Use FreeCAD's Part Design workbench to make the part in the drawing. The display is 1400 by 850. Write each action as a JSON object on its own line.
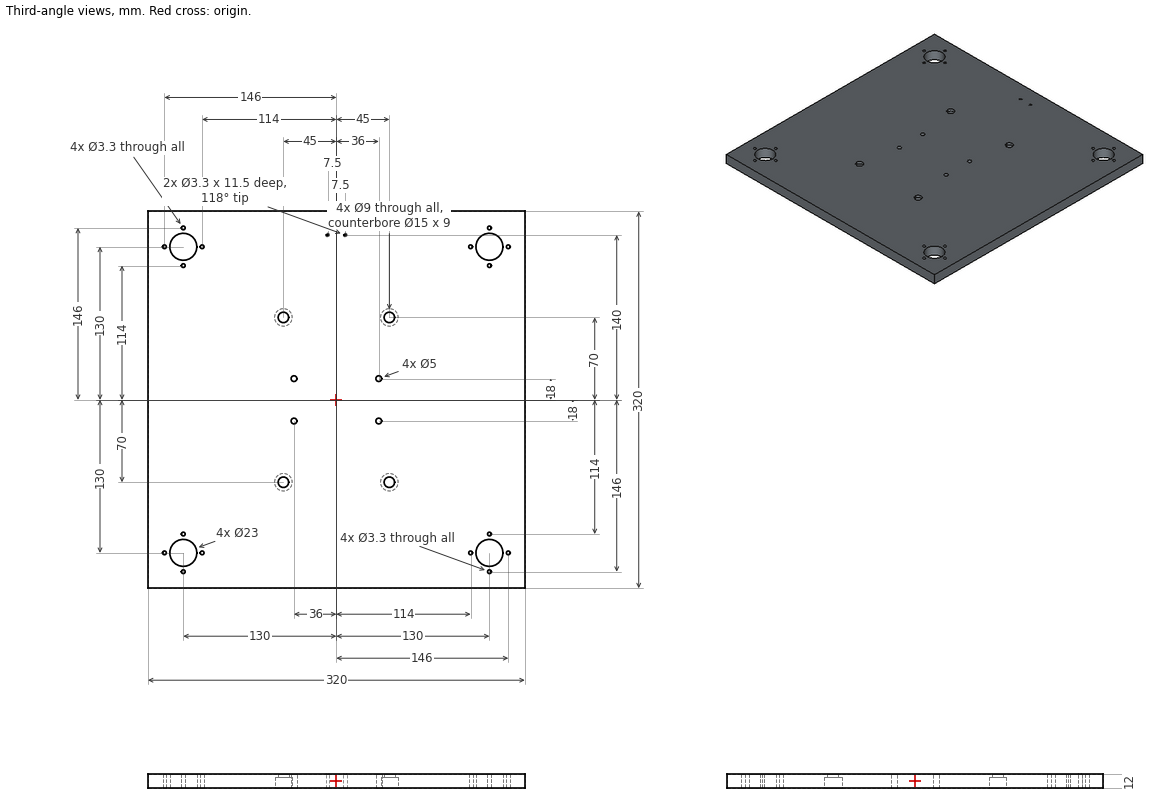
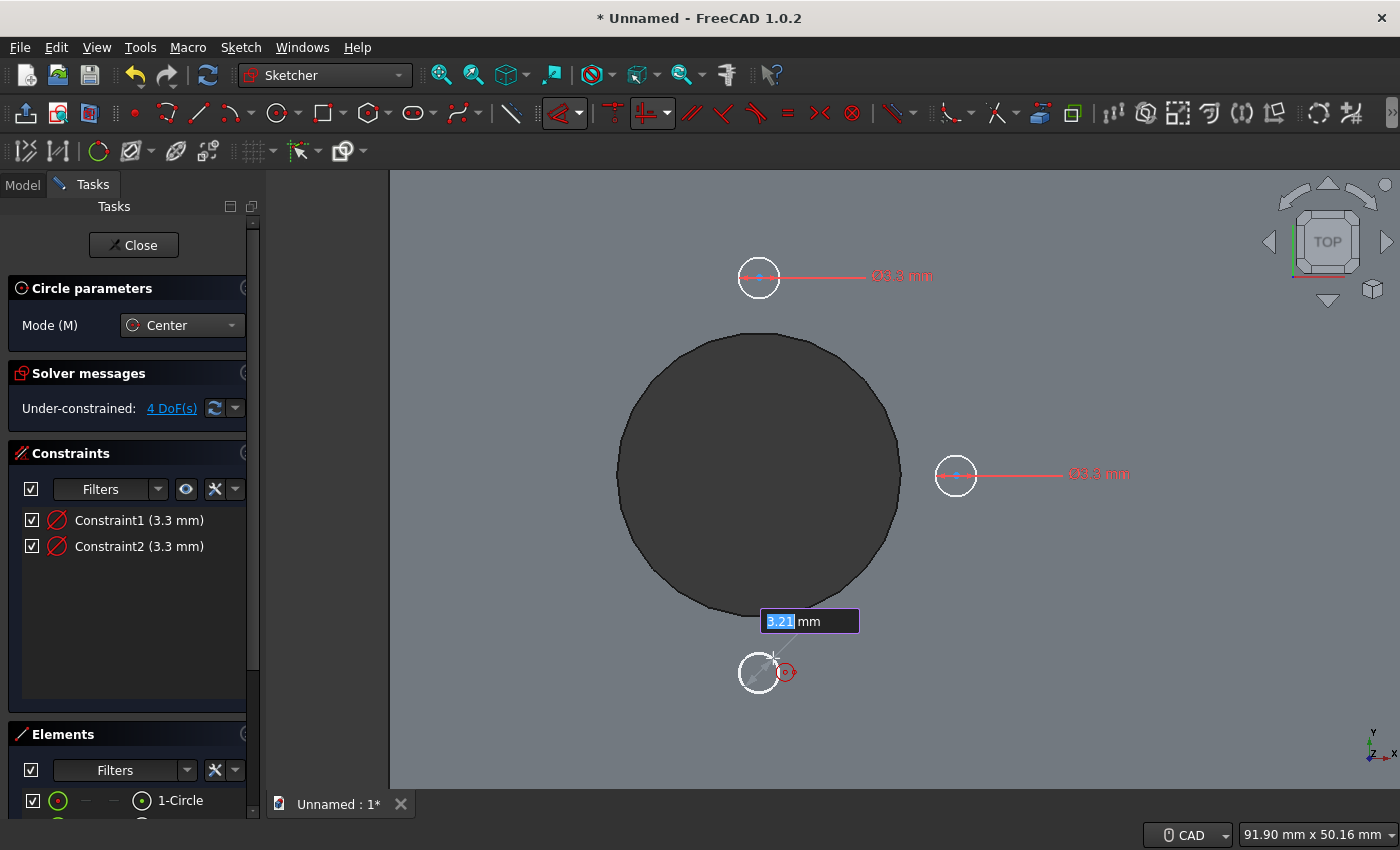
{"action": "type", "text": "3.3"}
{"action": "key", "text": "Return"}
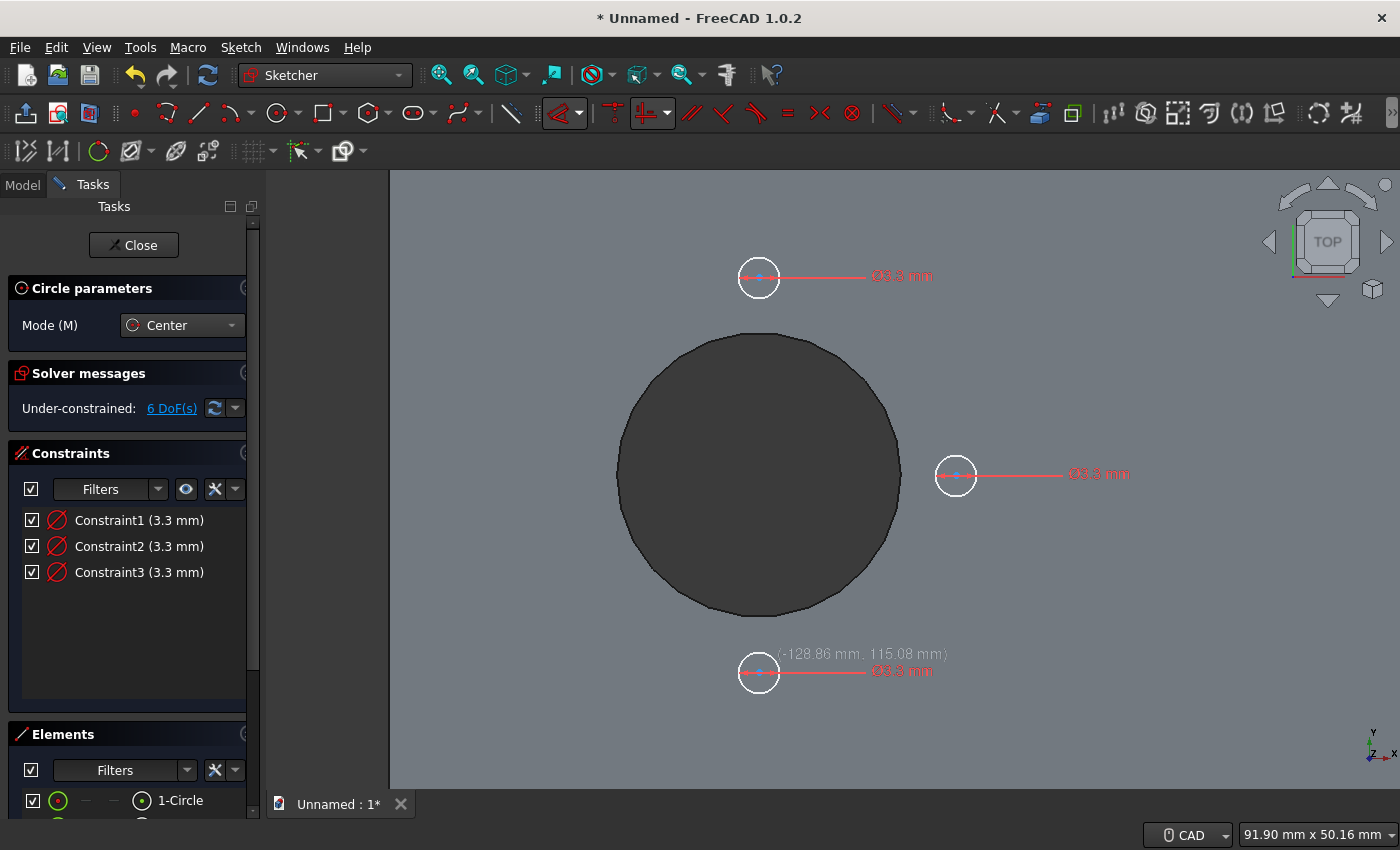
{"action": "left_click", "coordinate": [561, 475]}
{"action": "mouse_move", "coordinate": [576, 460]}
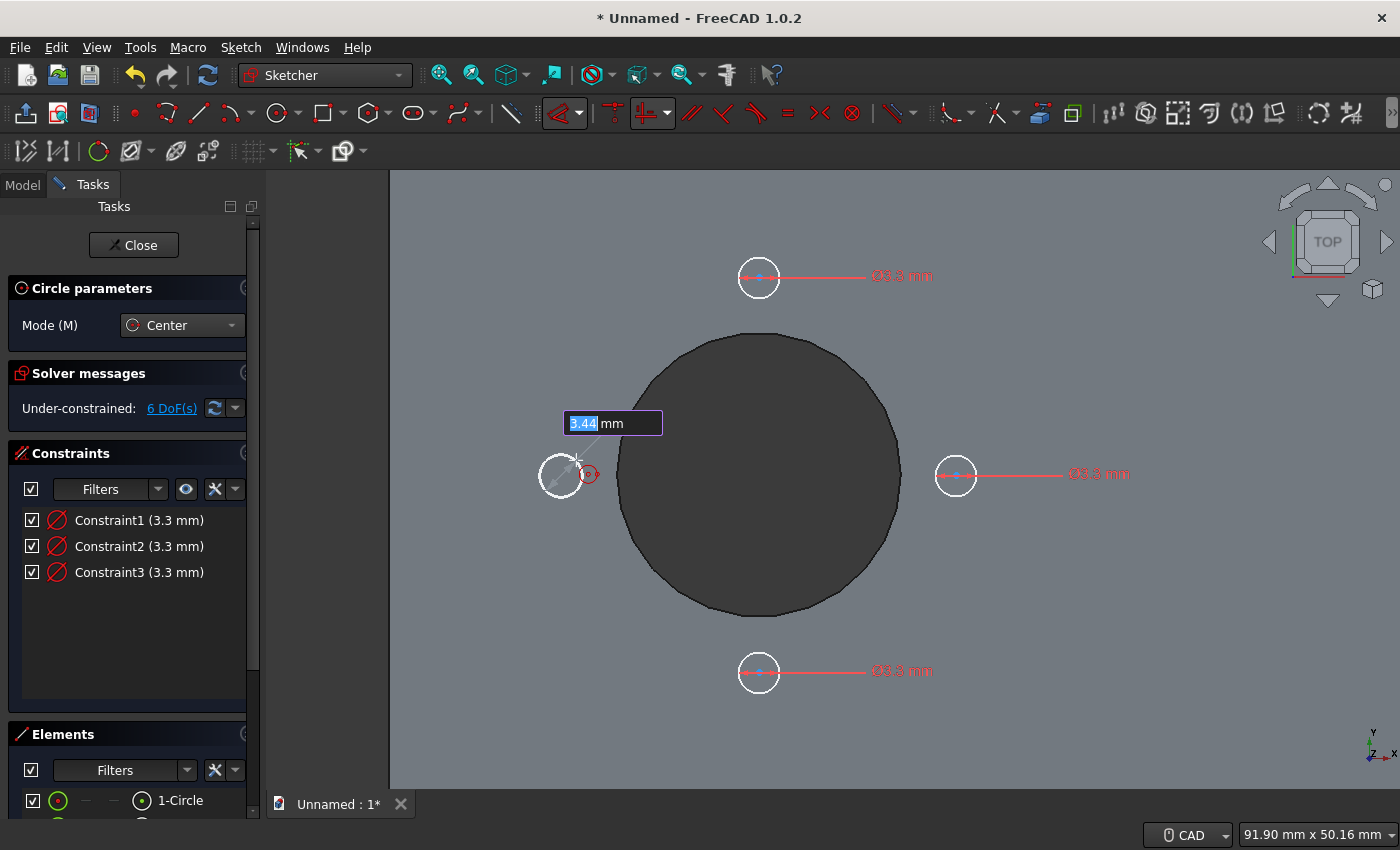
{"action": "type", "text": "3.3"}
{"action": "key", "text": "Return"}
{"action": "key", "text": "Escape"}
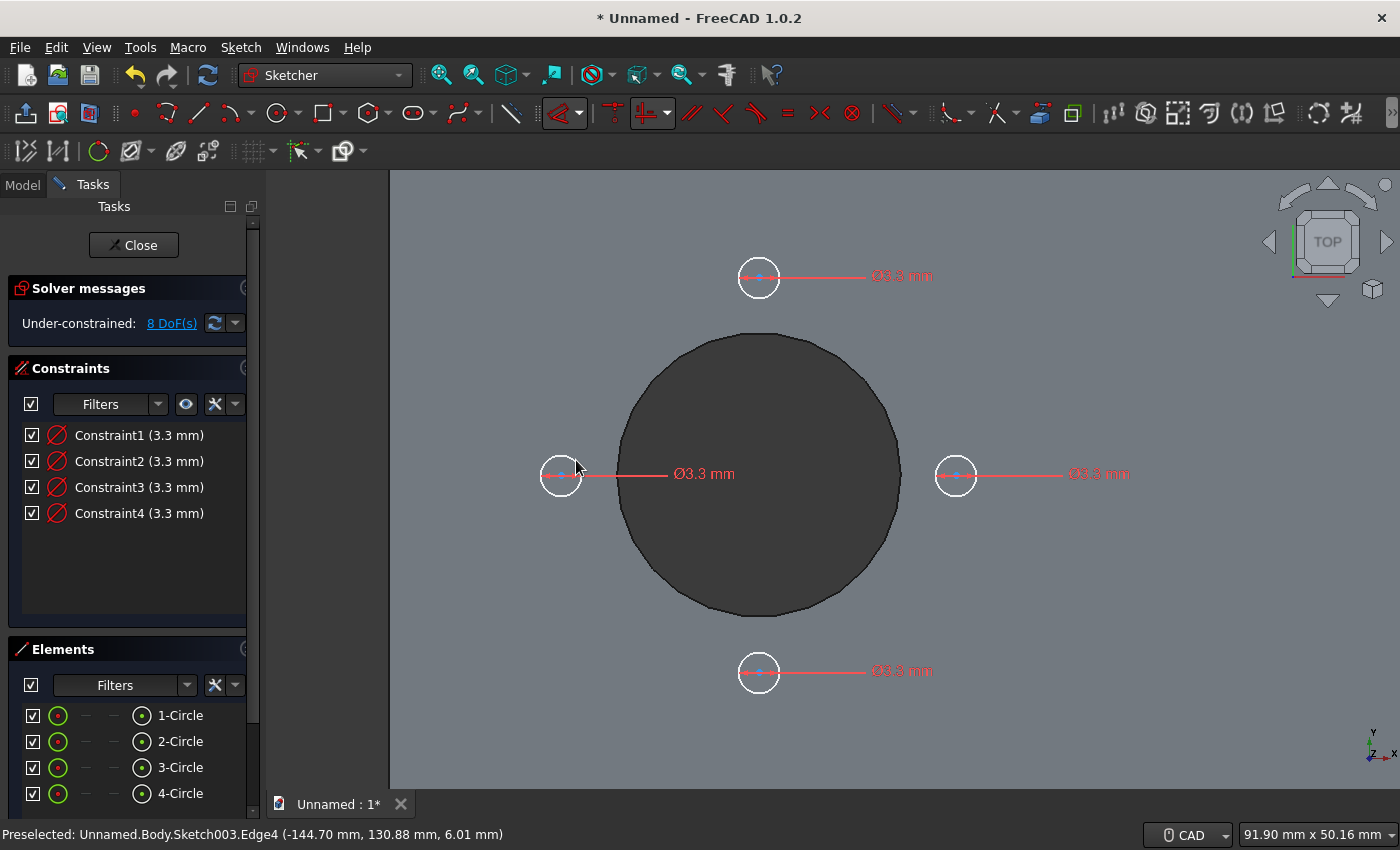
{"action": "left_click", "coordinate": [759, 278]}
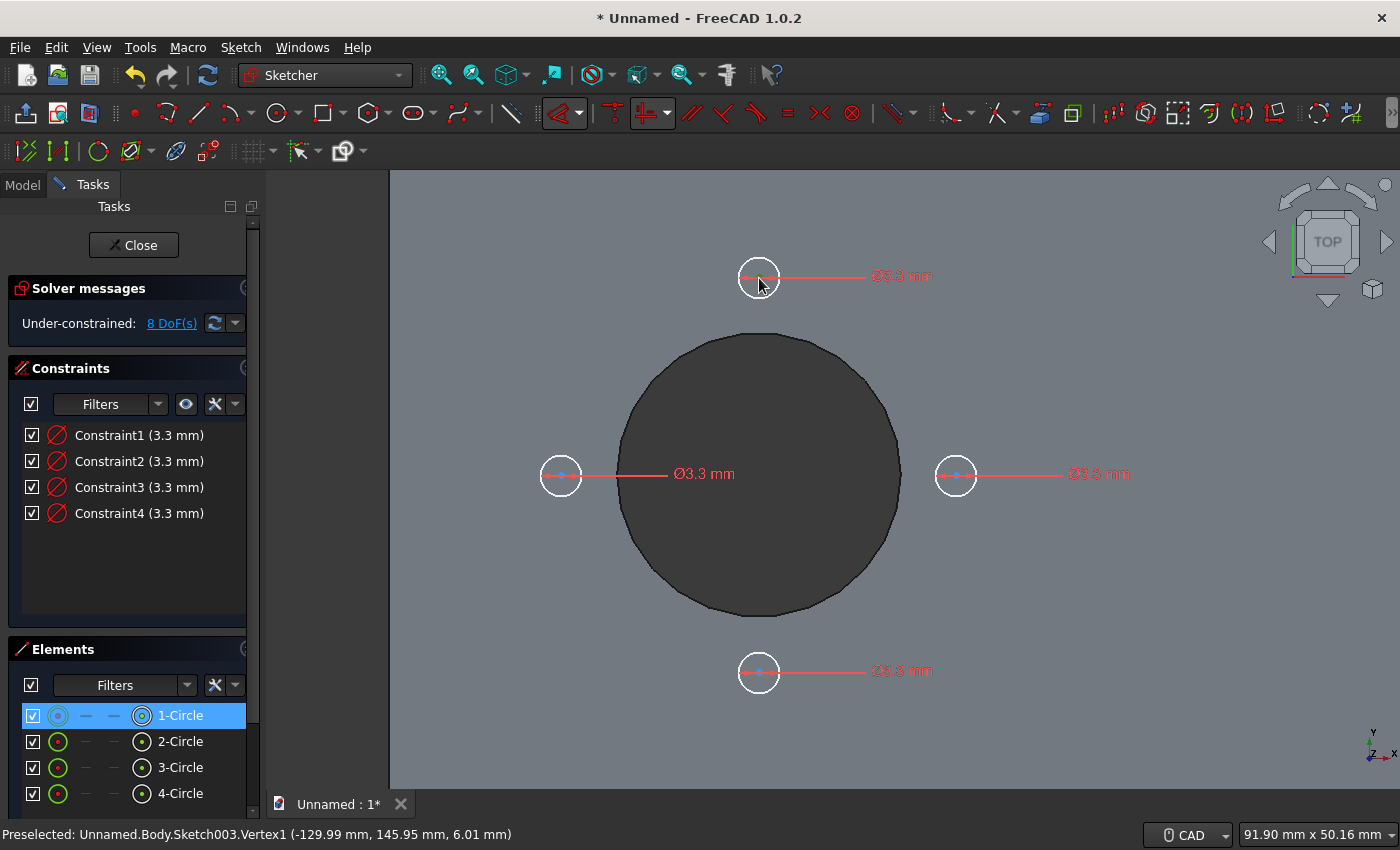
{"action": "left_click", "coordinate": [759, 673]}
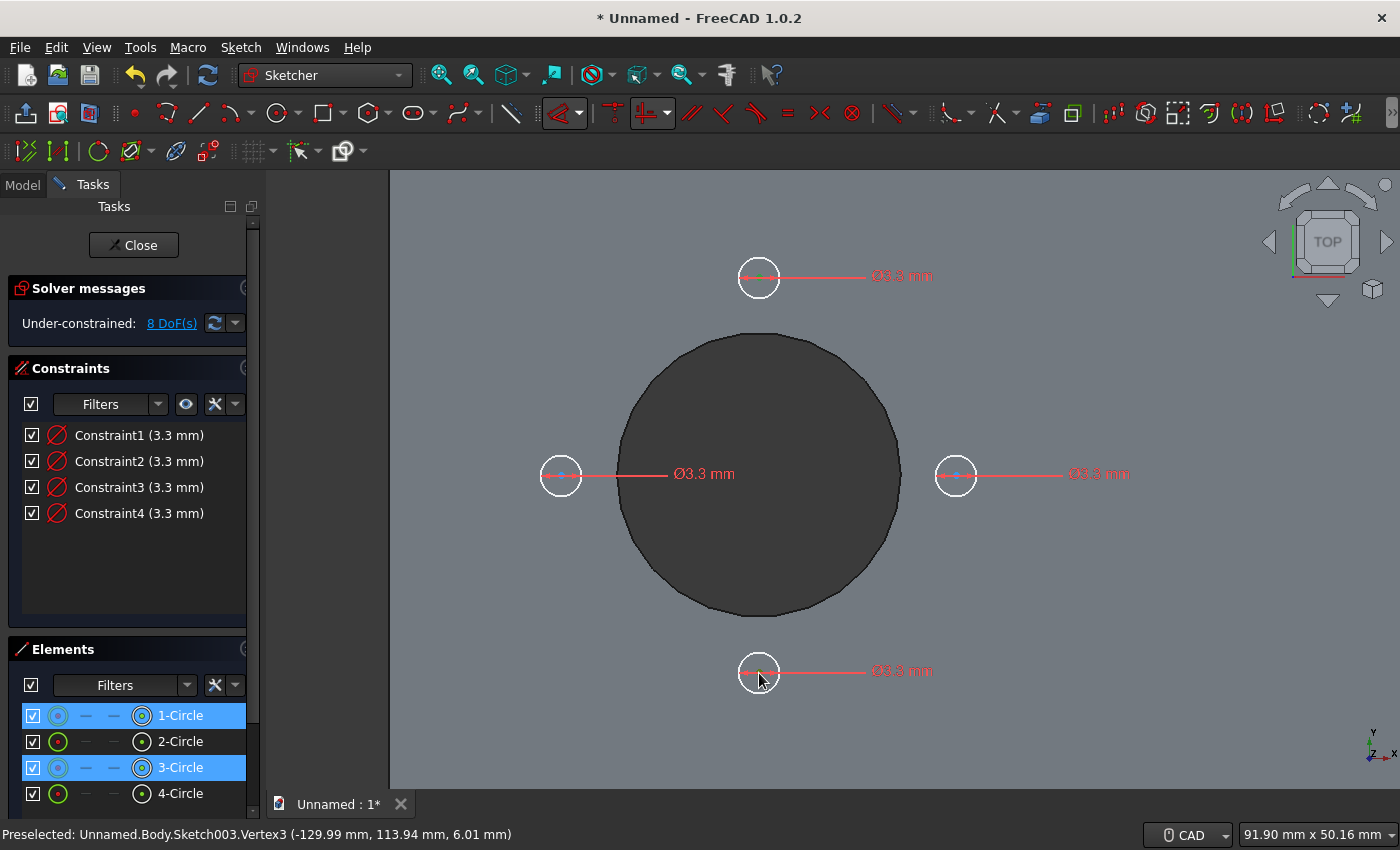
{"action": "left_click", "coordinate": [670, 114]}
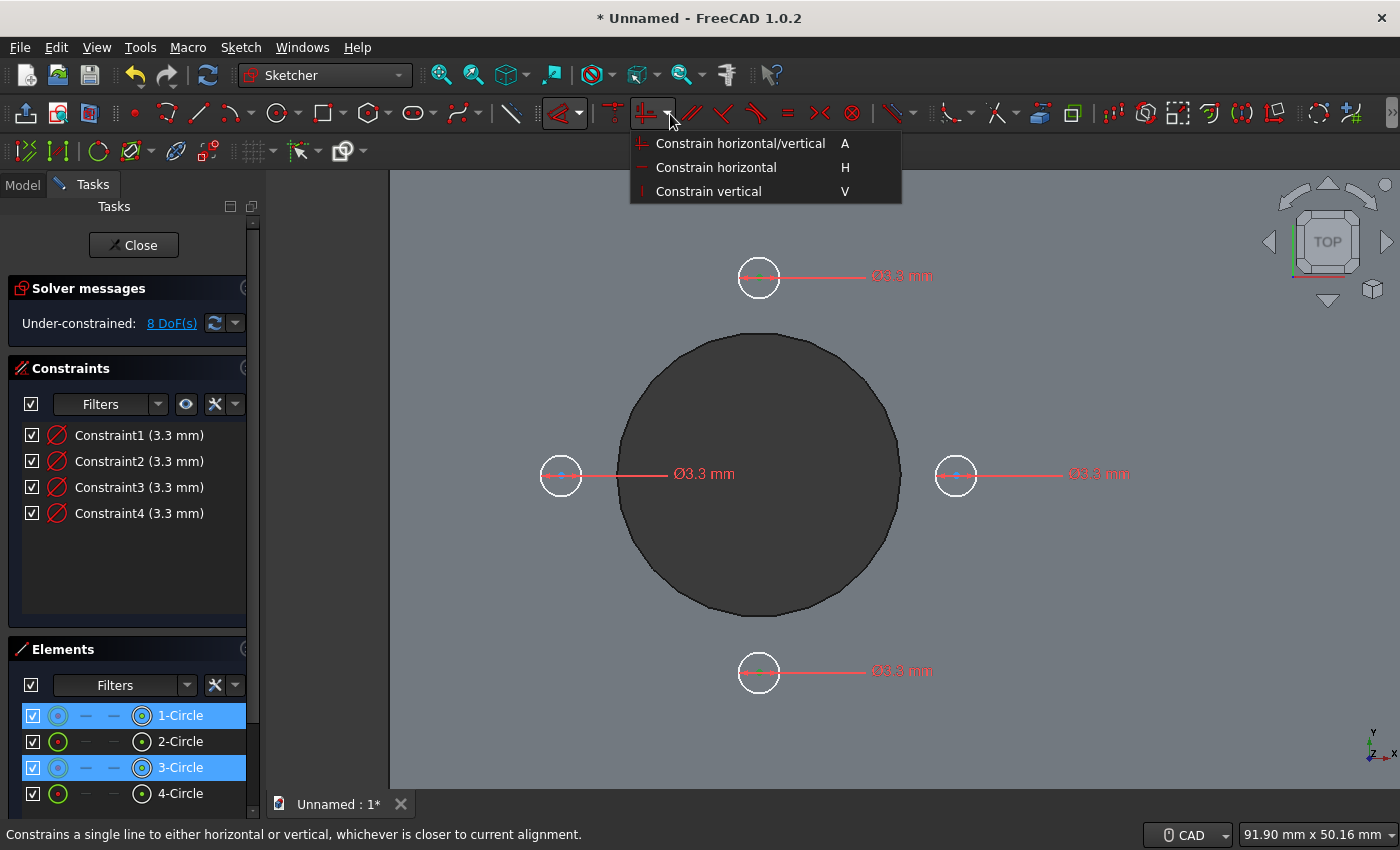
{"action": "left_click", "coordinate": [766, 191]}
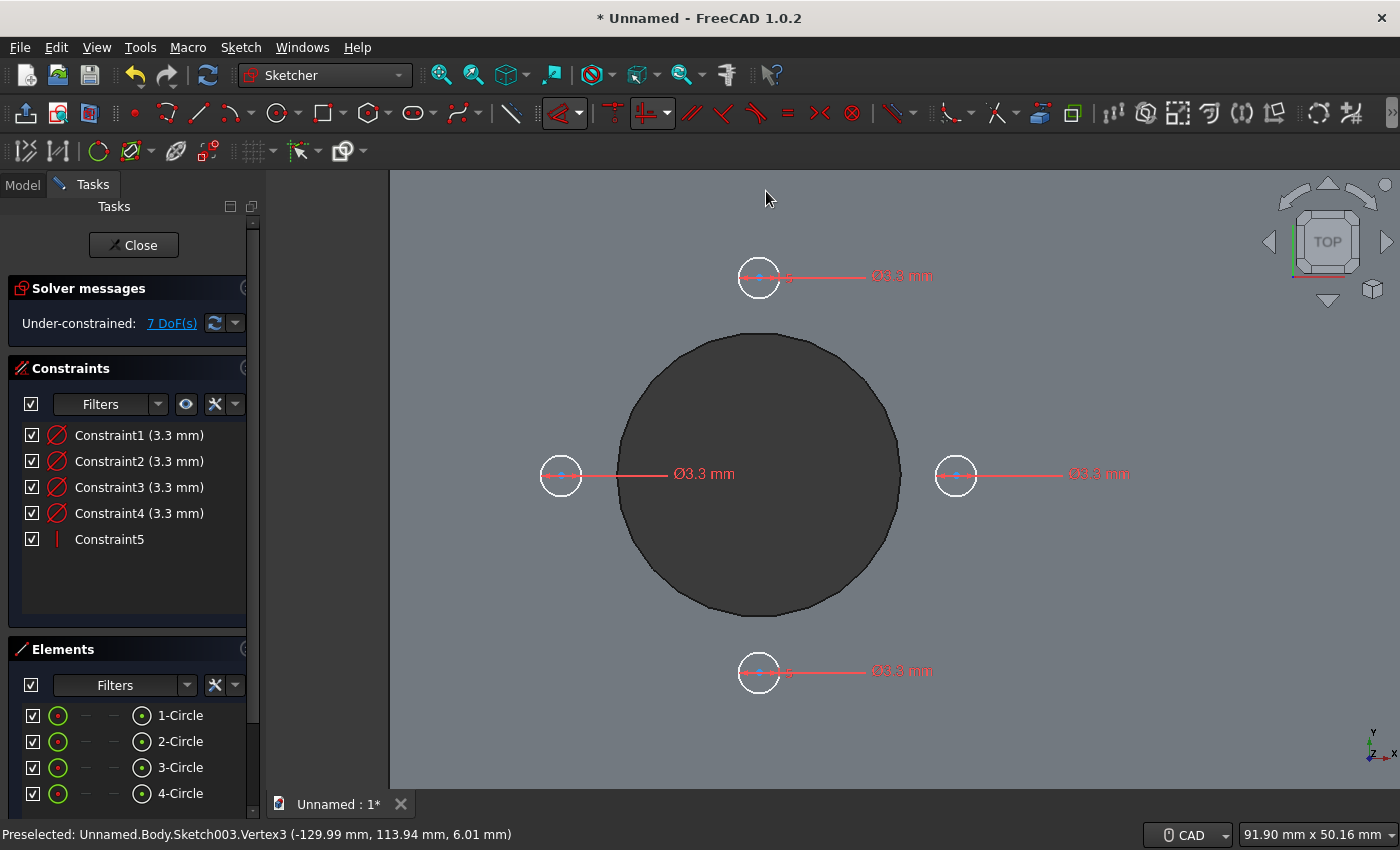
{"action": "left_click", "coordinate": [956, 476]}